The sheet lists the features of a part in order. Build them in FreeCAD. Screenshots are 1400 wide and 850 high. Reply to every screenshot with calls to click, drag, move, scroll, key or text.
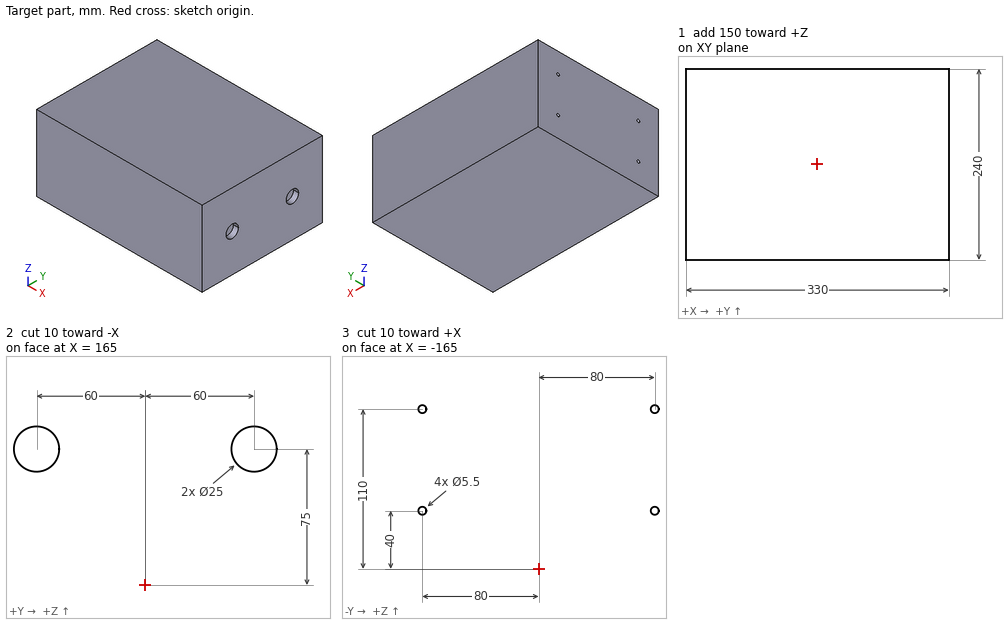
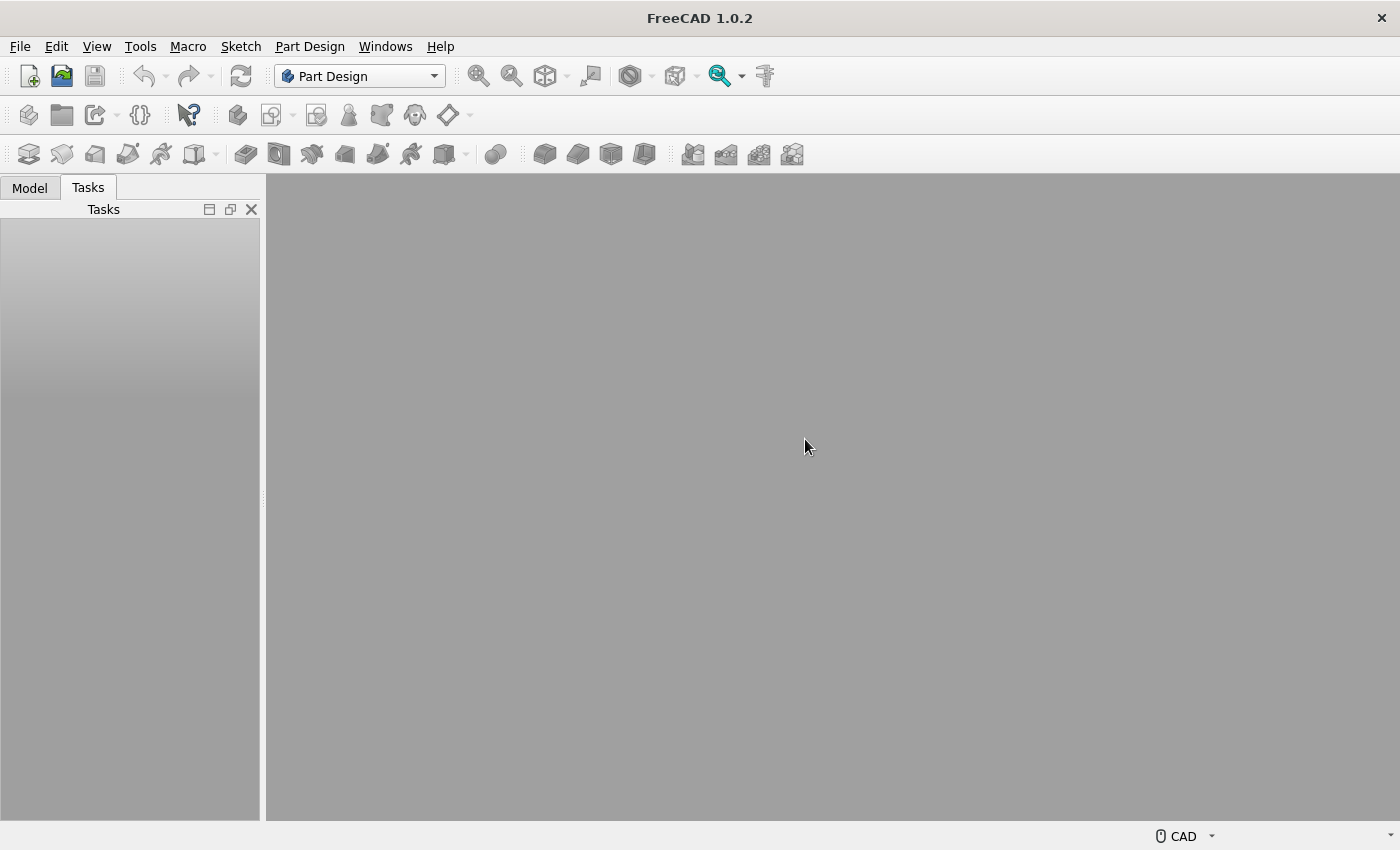
click(29, 76)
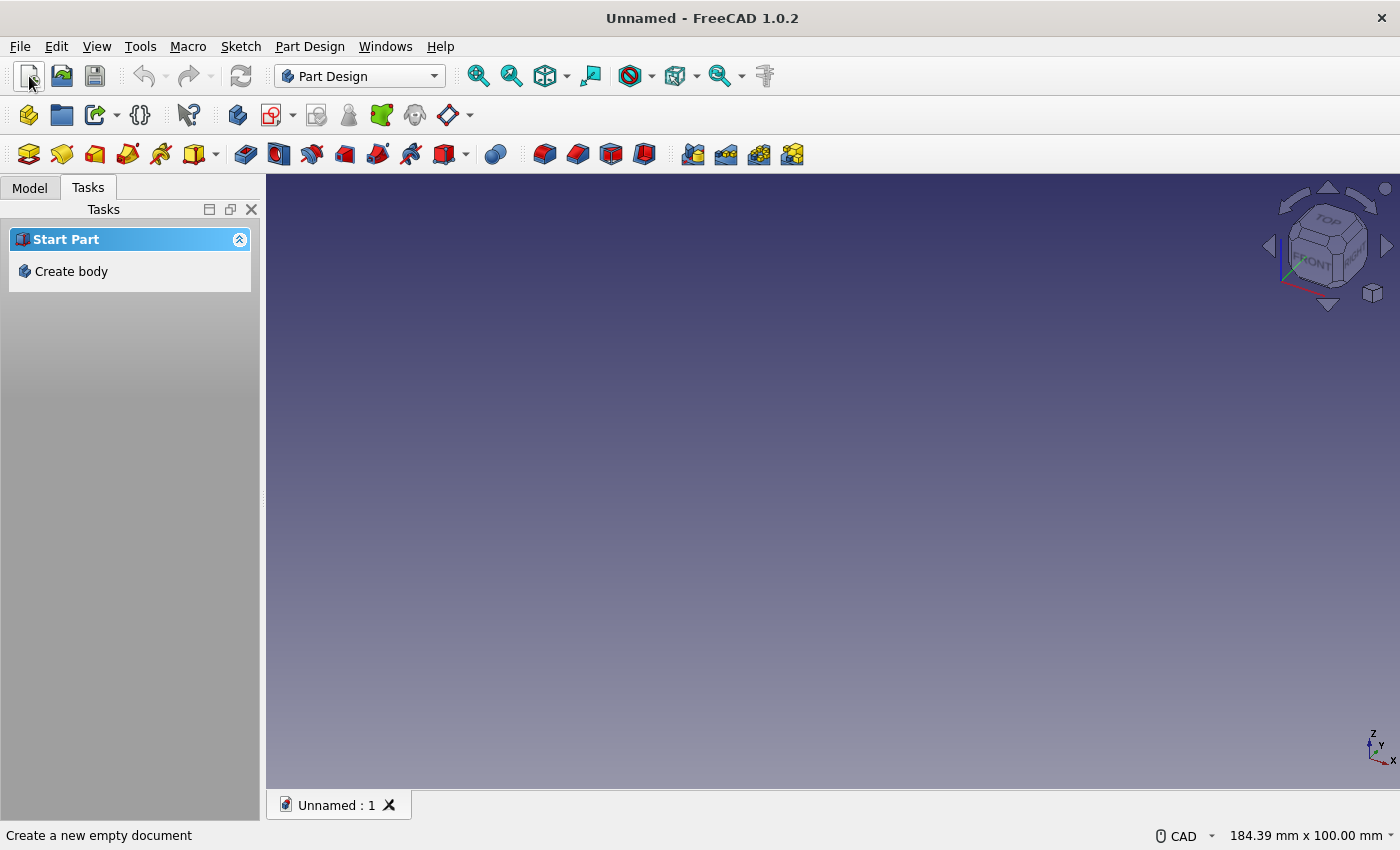
click(270, 116)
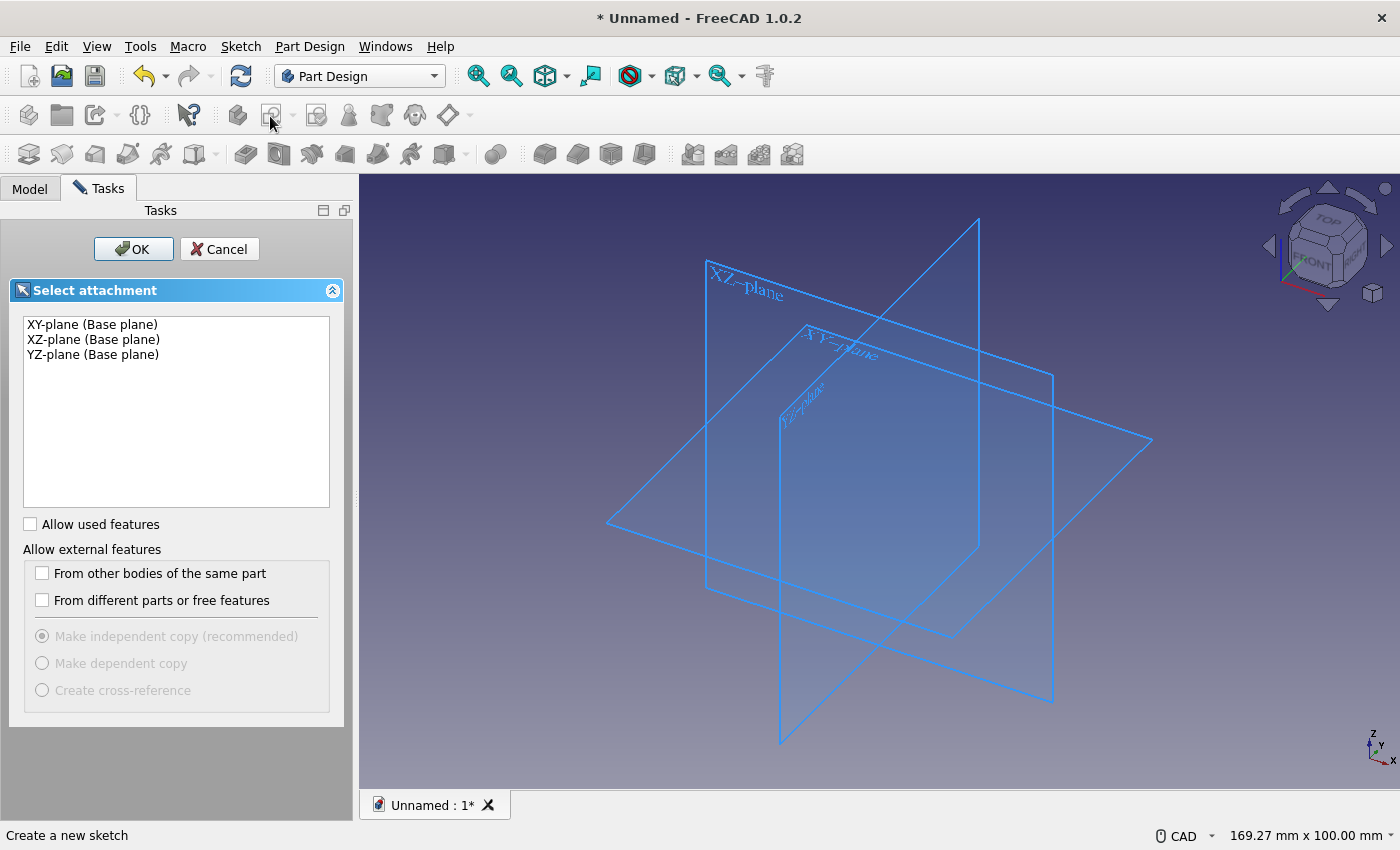
click(84, 324)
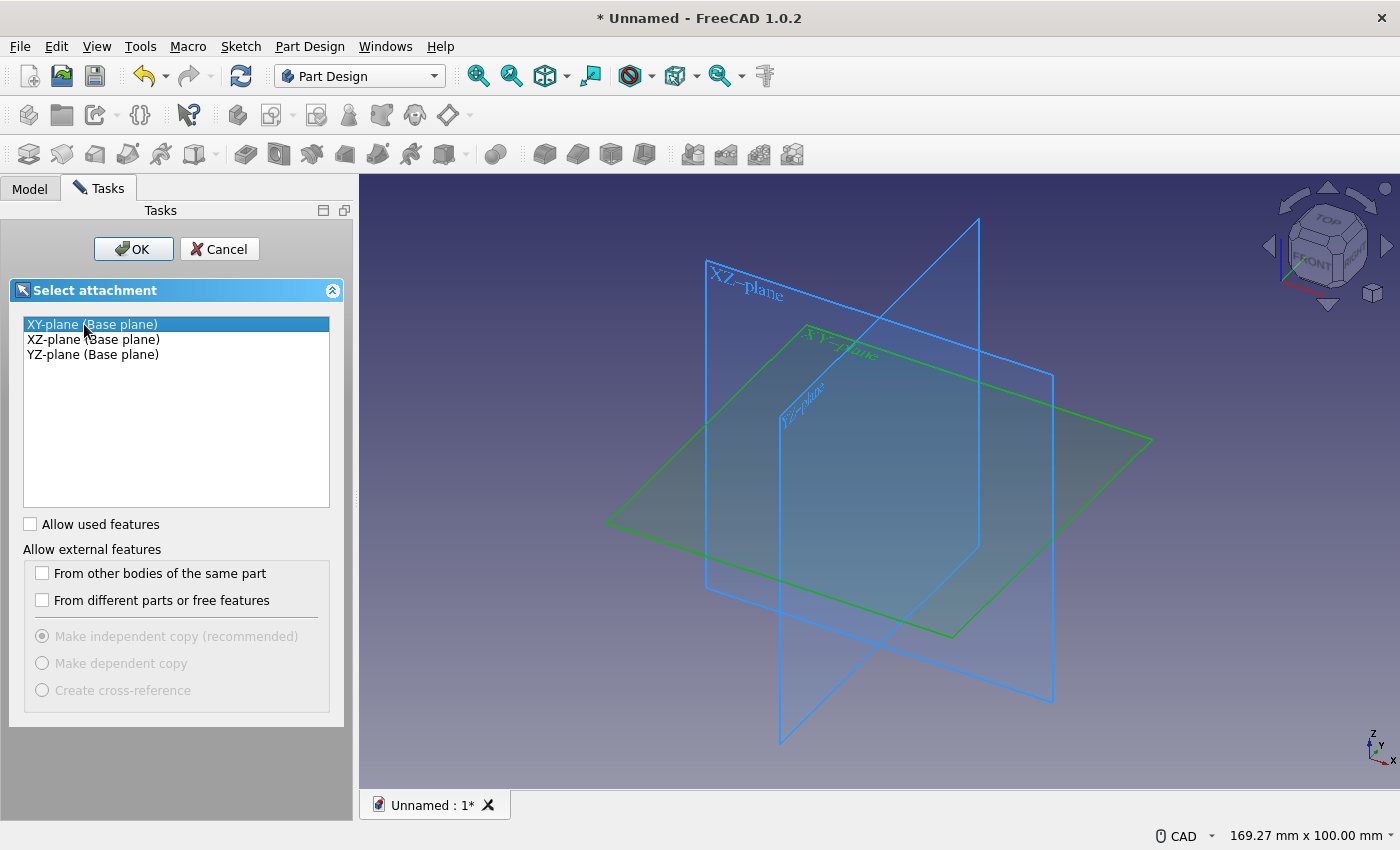
click(134, 249)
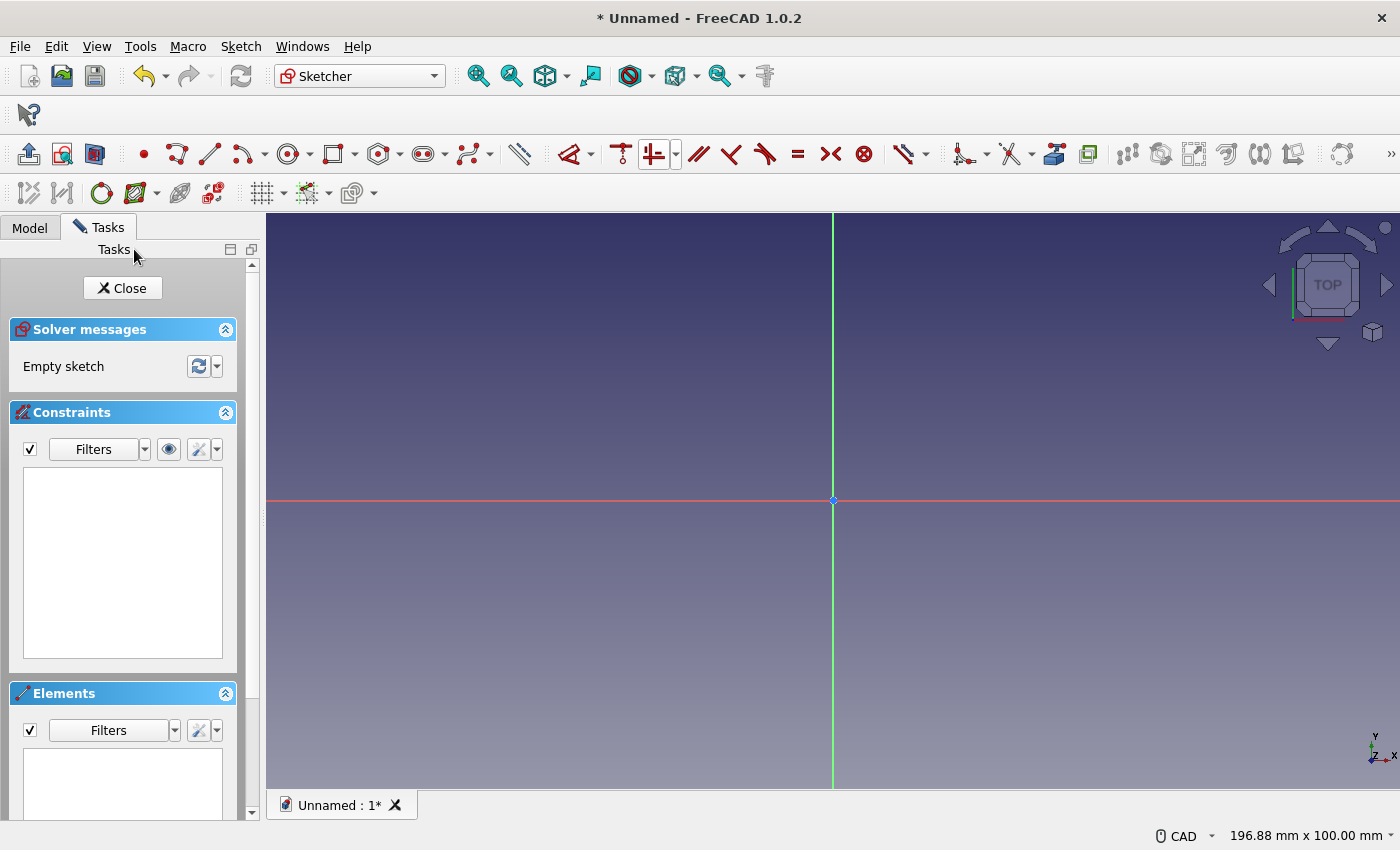
scroll(742, 501, down, 7)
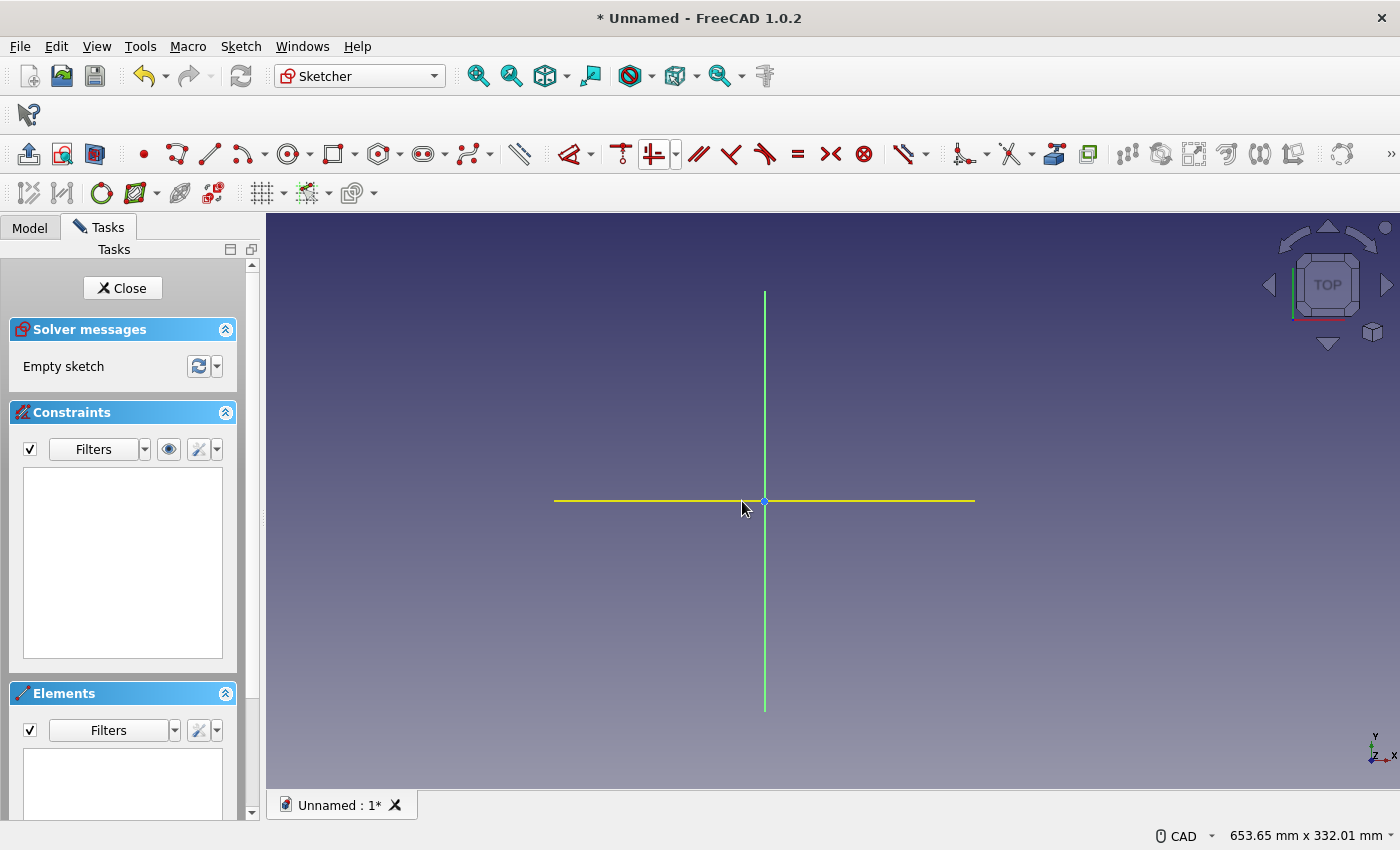
click(354, 154)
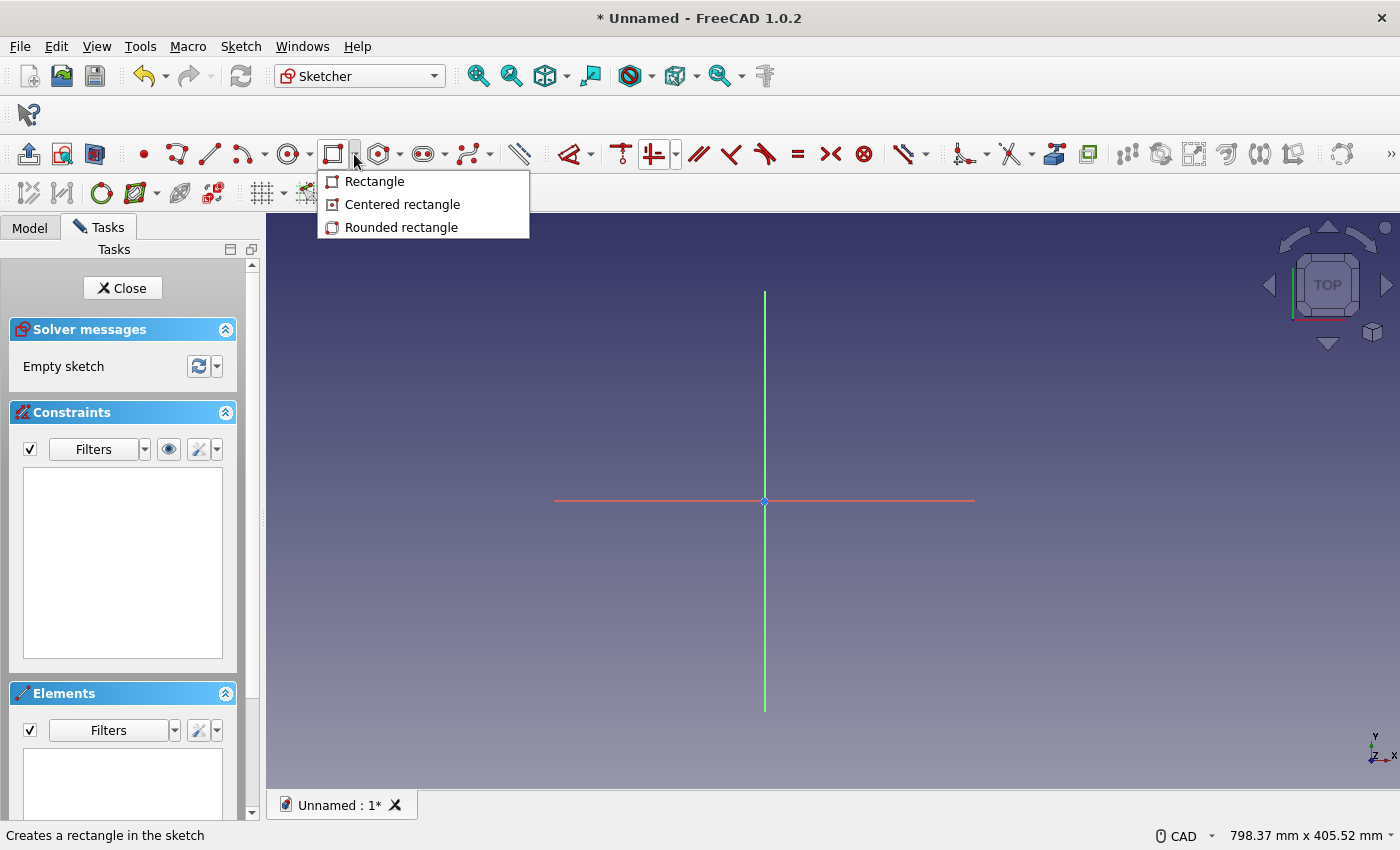
click(424, 204)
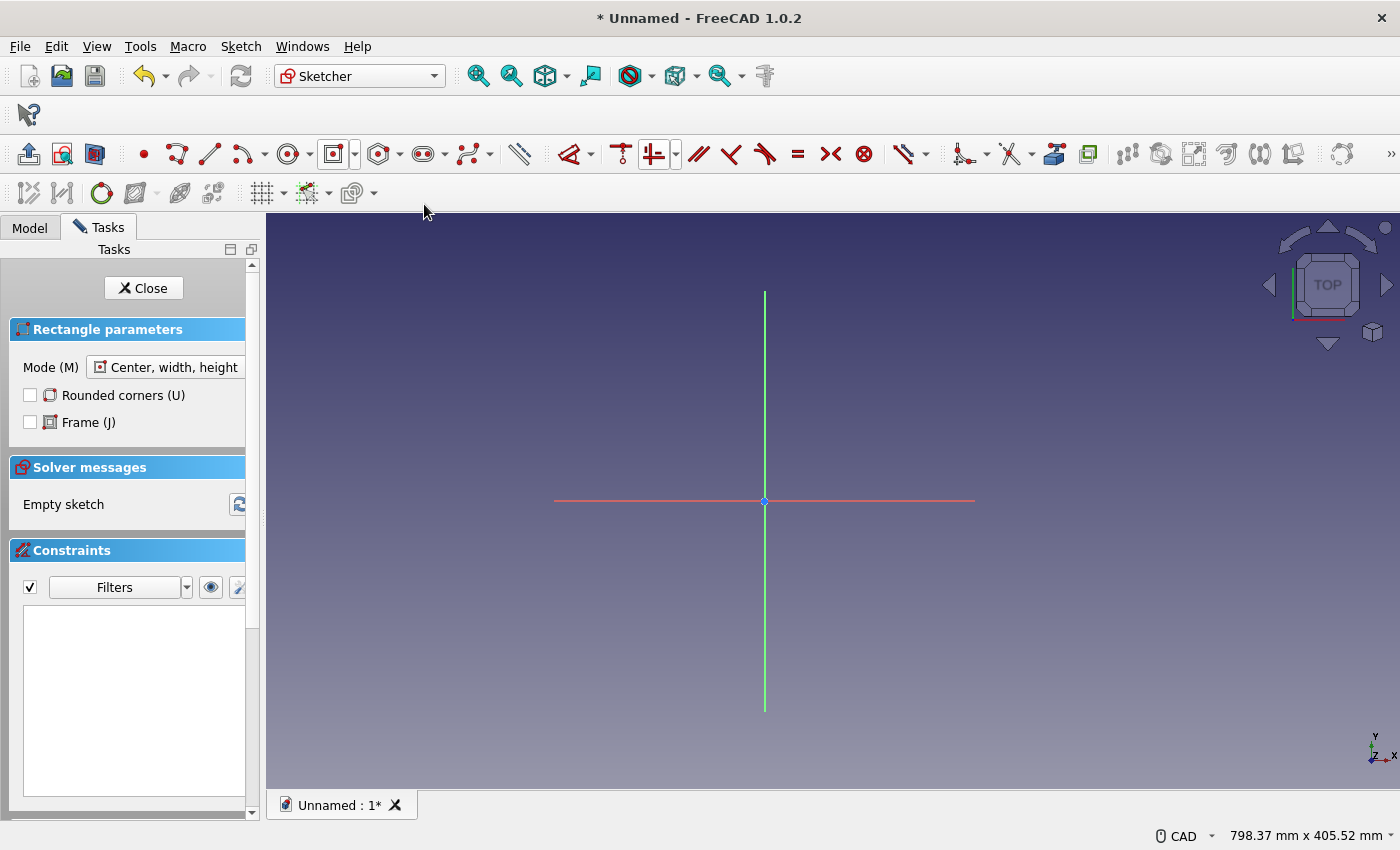
click(765, 501)
move(999, 331)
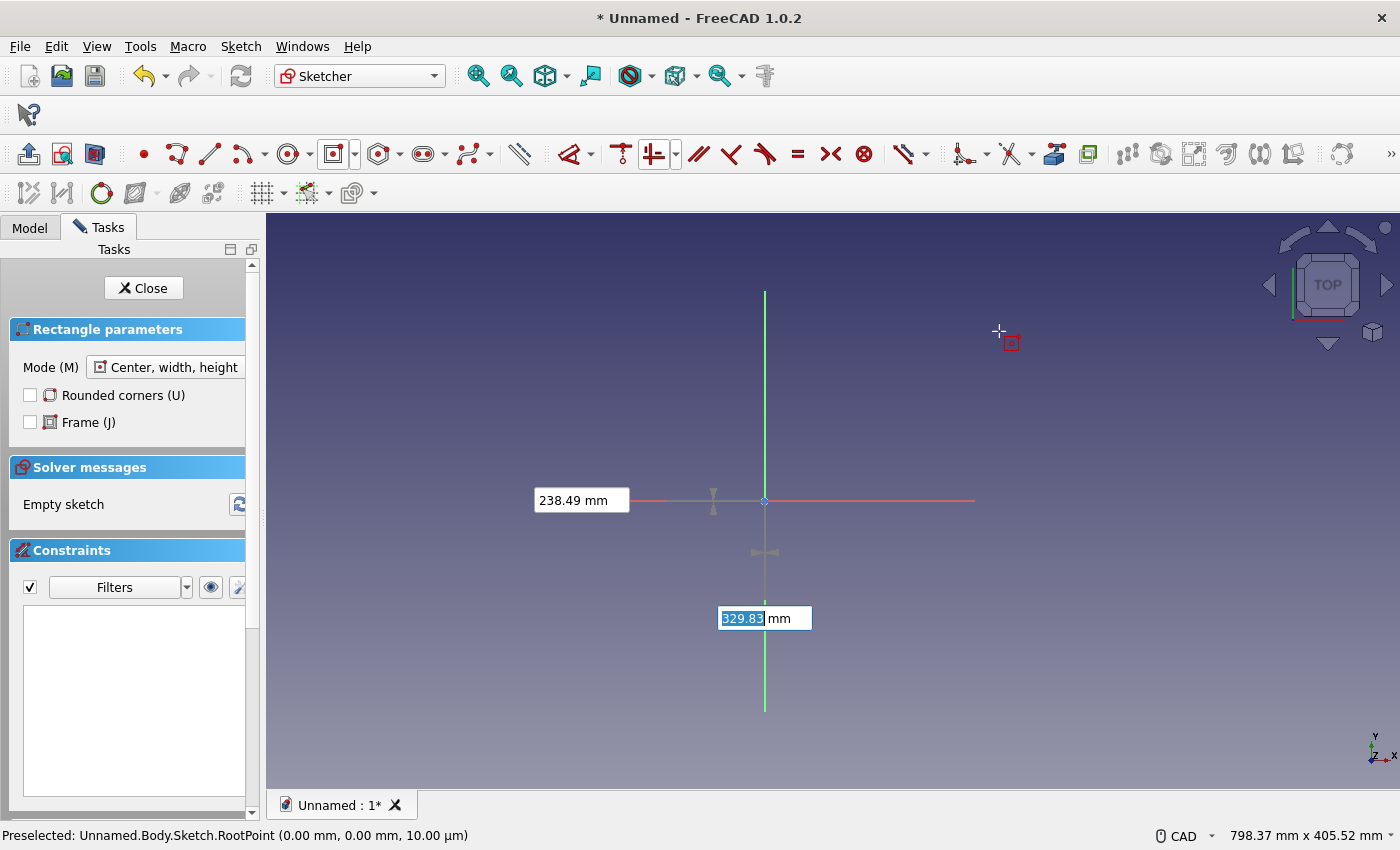
text(330)
key(Tab)
text(240)
key(Return)
key(Escape)